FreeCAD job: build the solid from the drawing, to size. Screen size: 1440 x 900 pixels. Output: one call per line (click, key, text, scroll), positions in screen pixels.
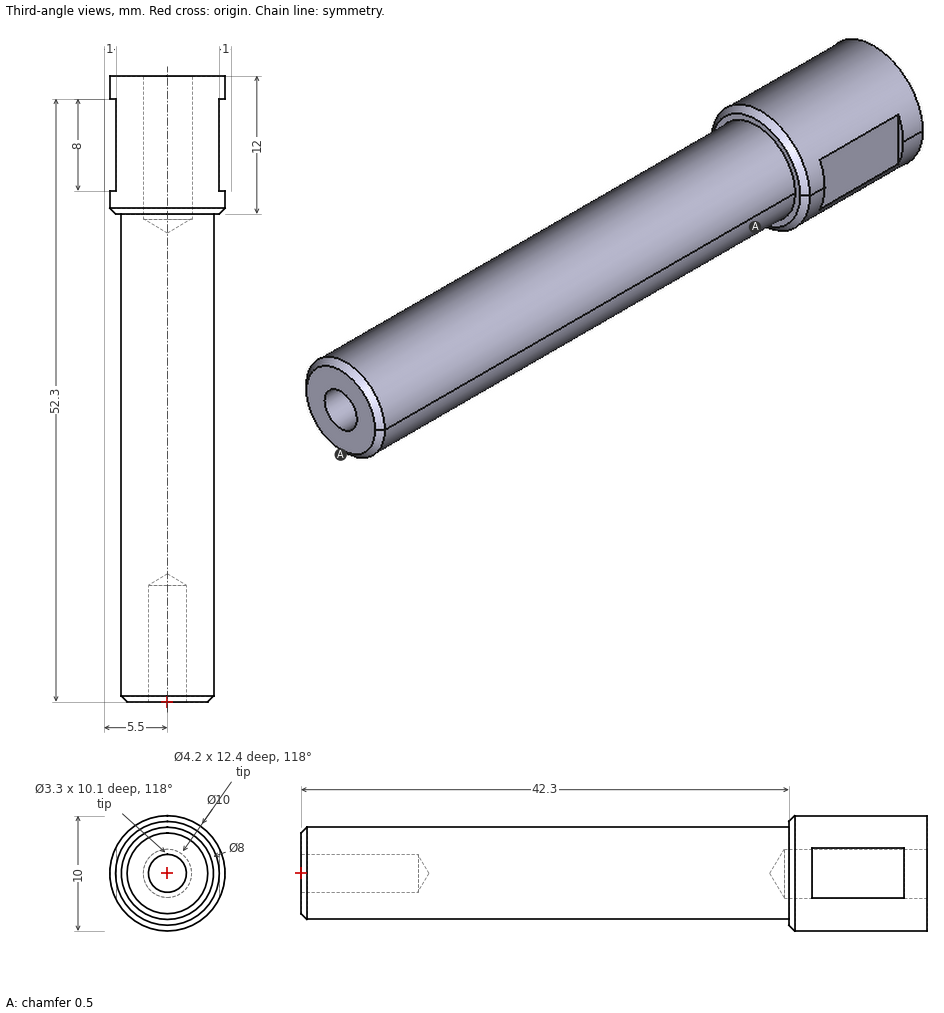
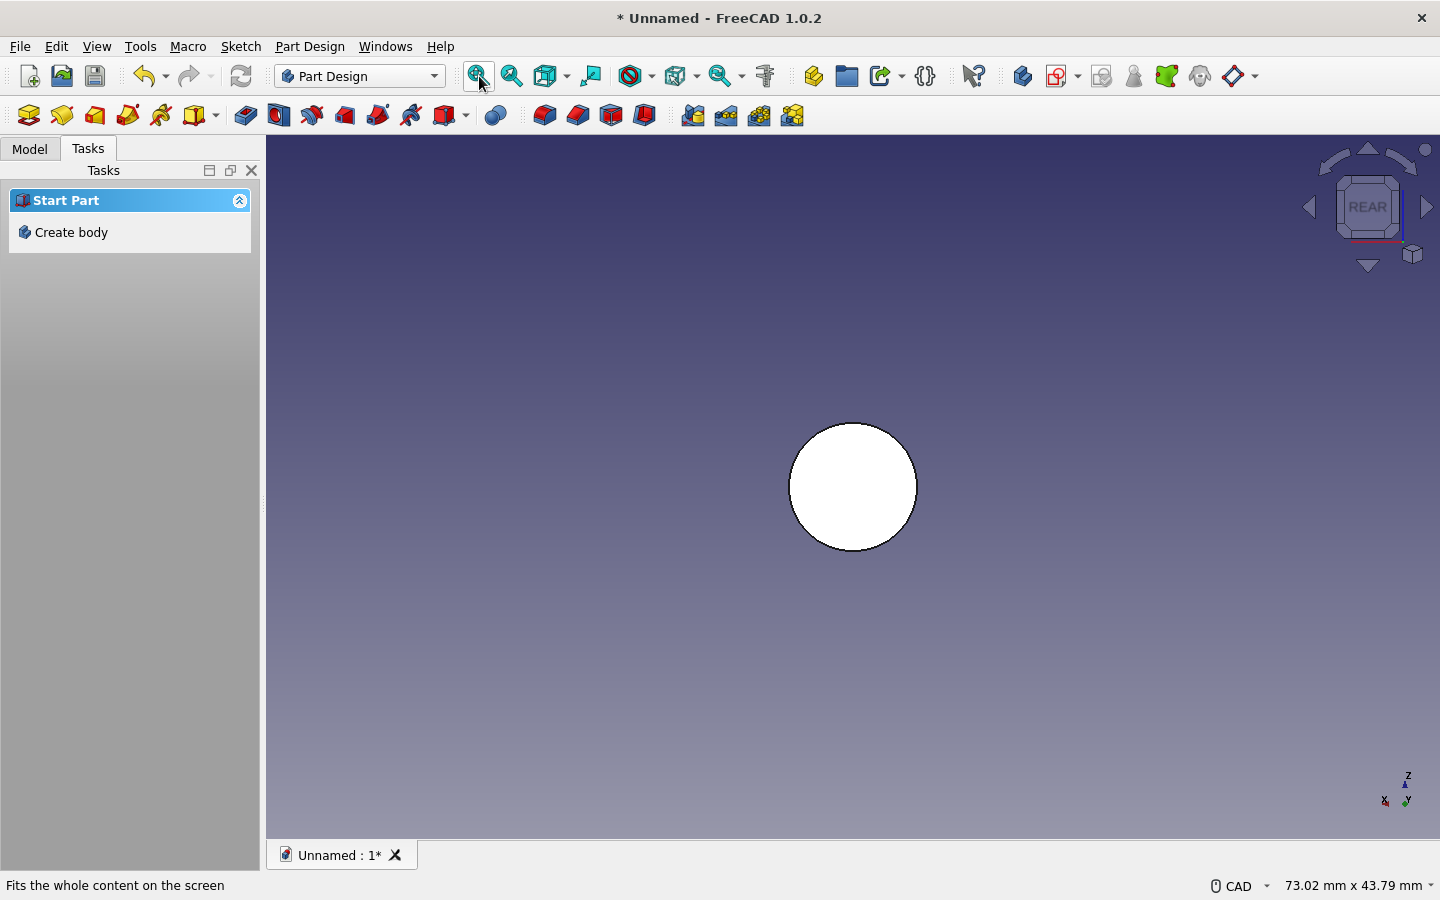
click(853, 486)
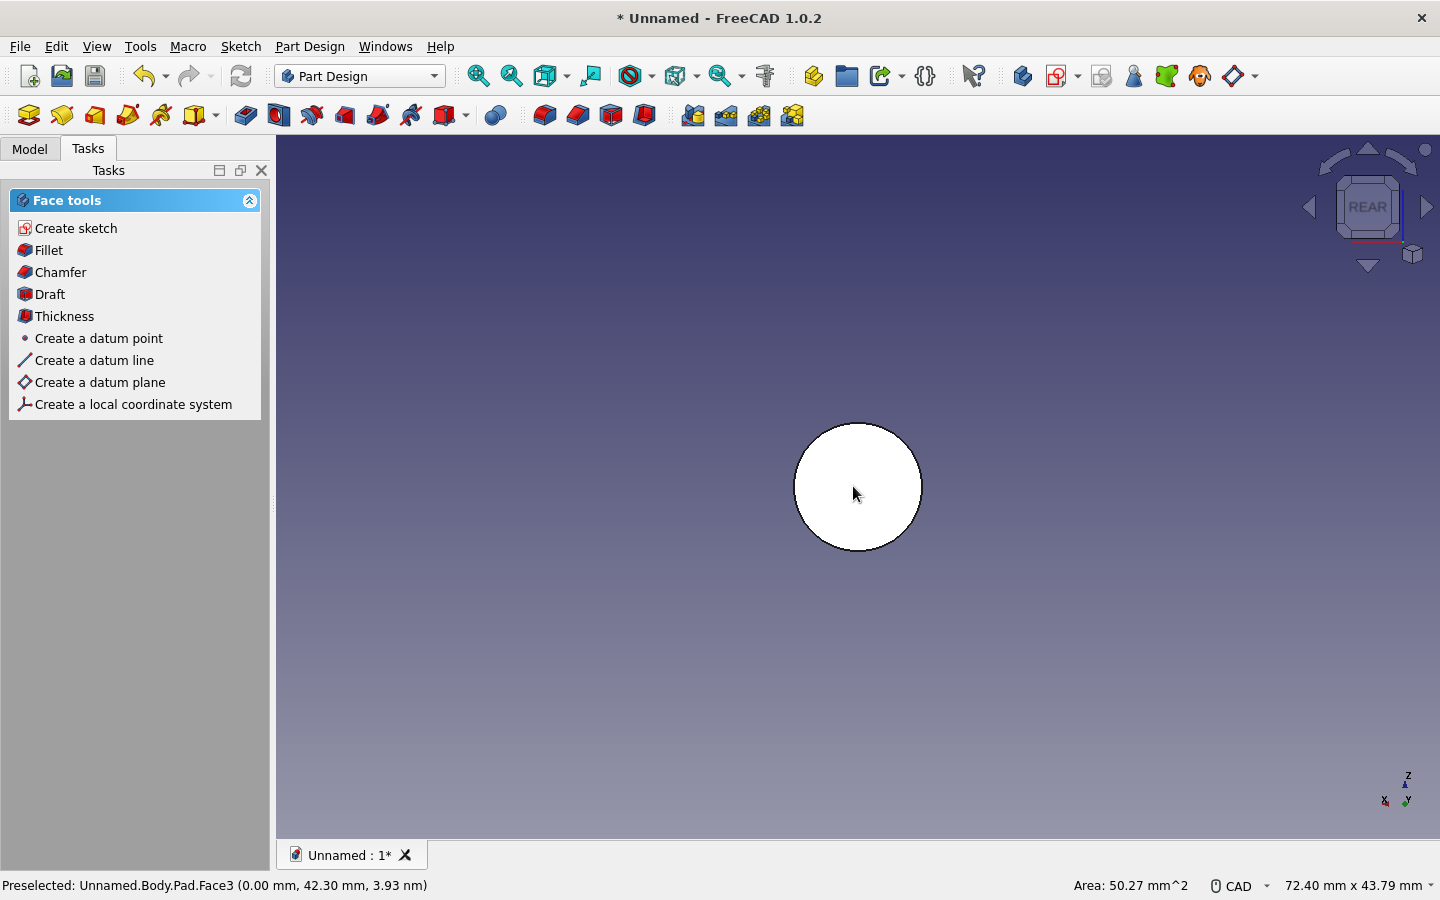
click(1056, 76)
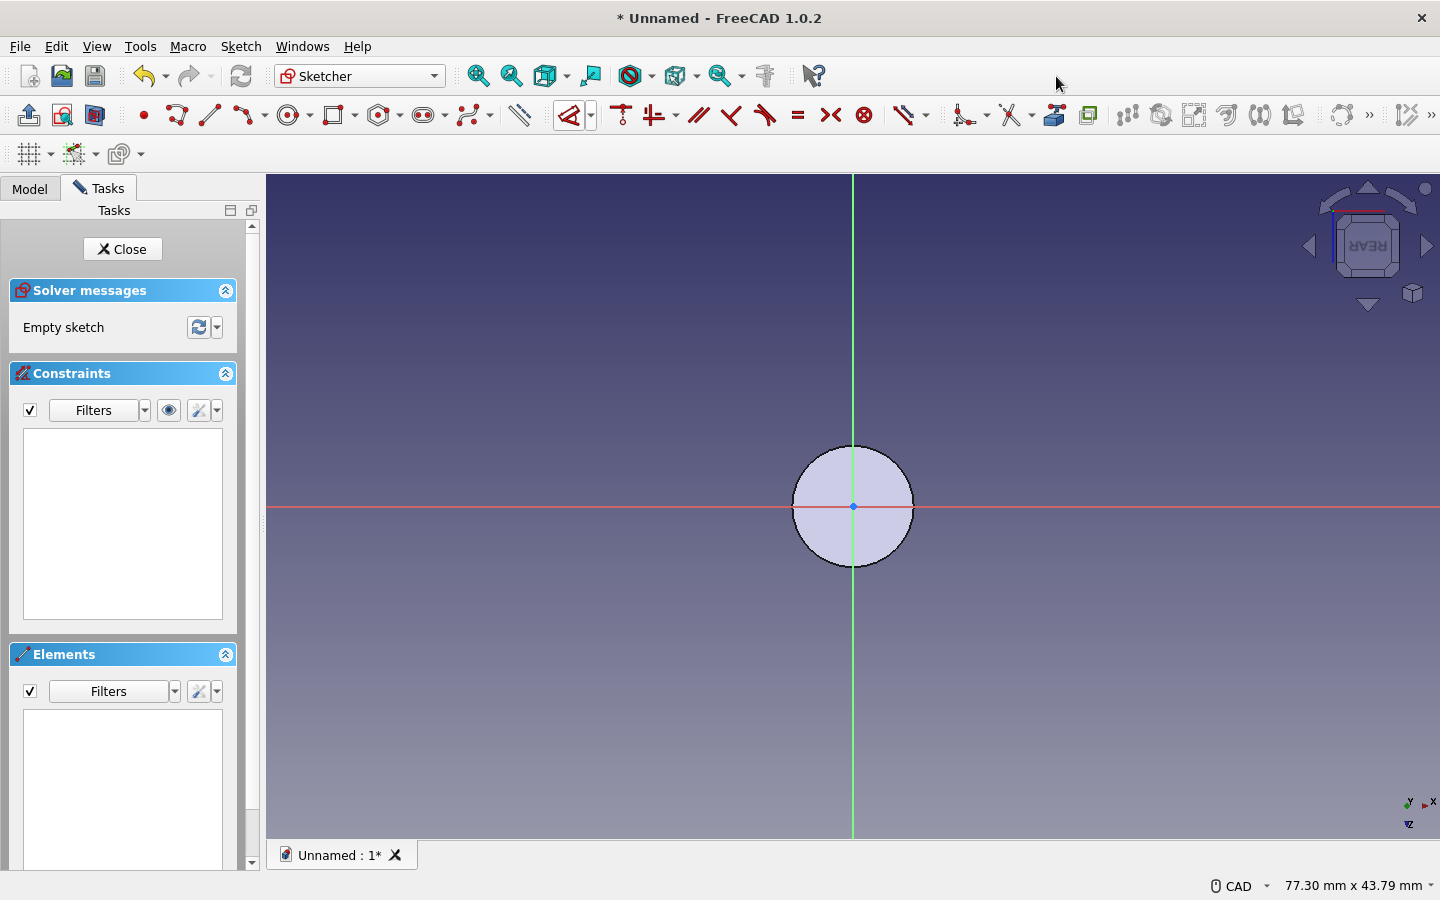
scroll(893, 506, up, 5)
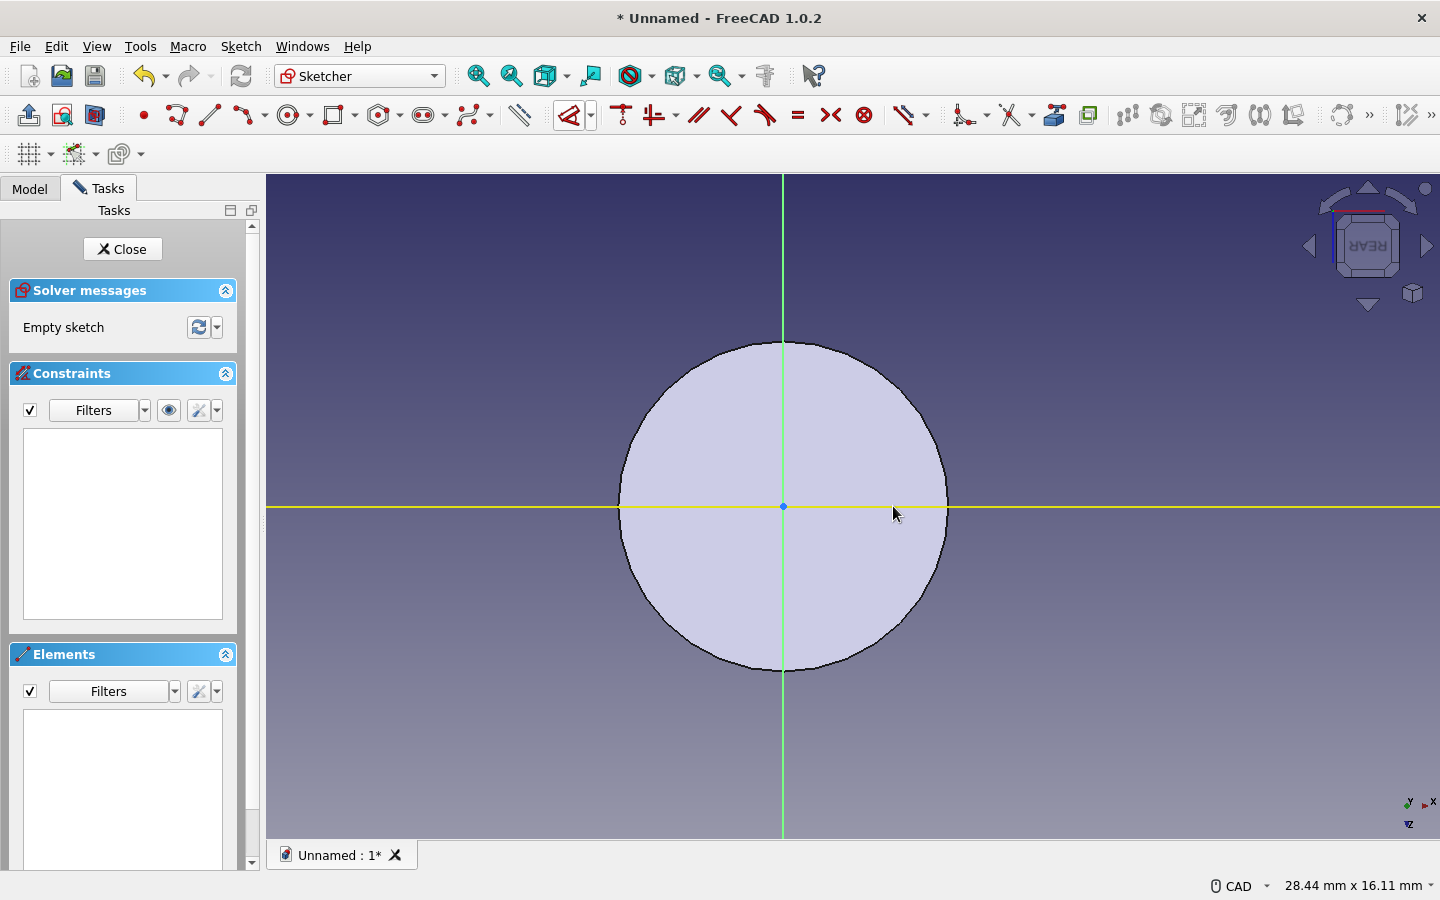
key(g)
key(c)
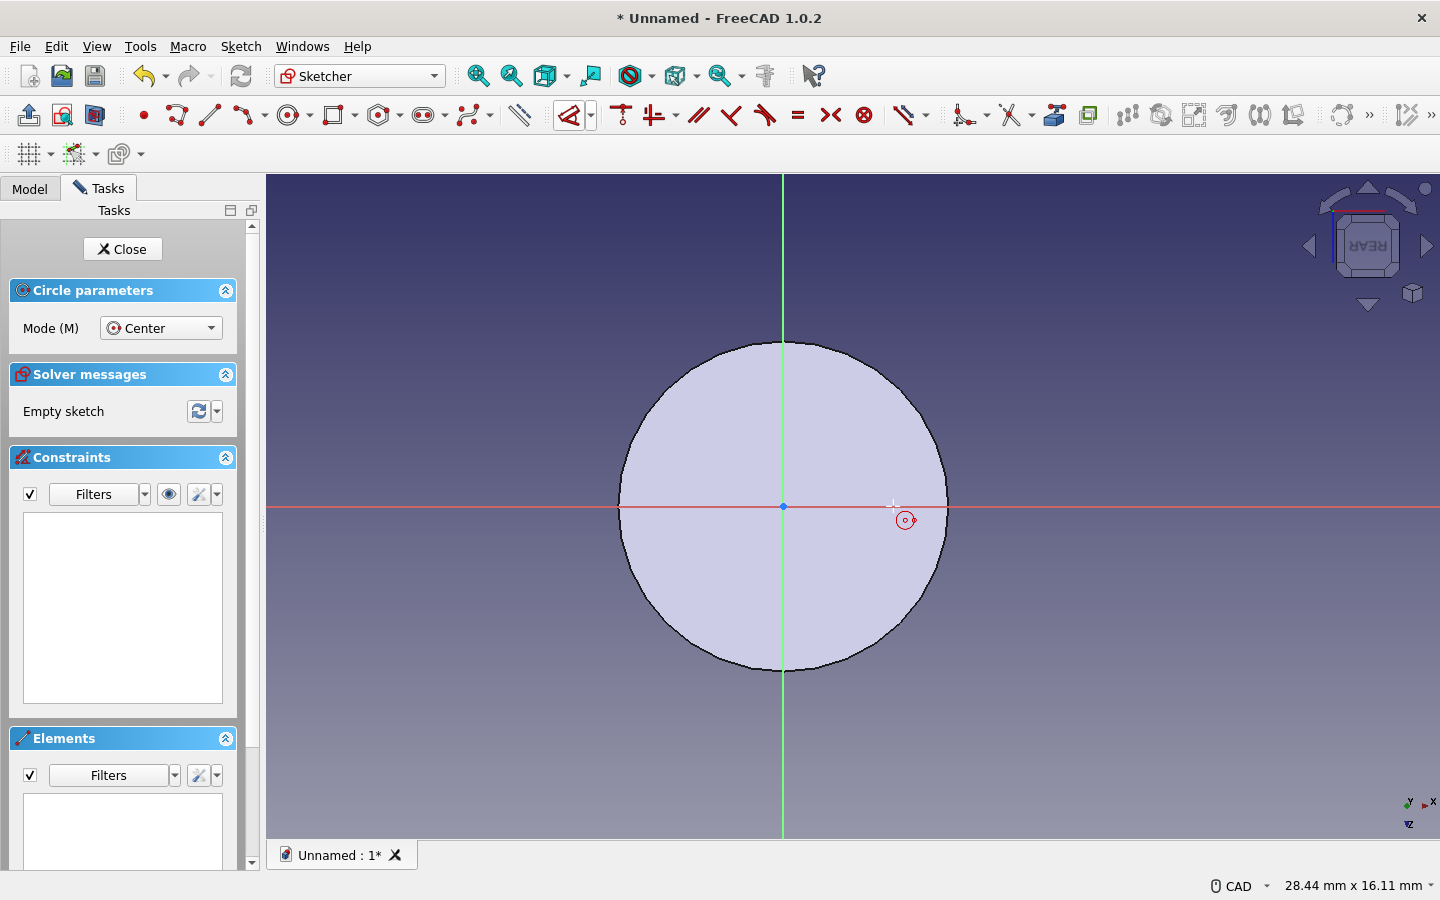
click(783, 506)
move(929, 361)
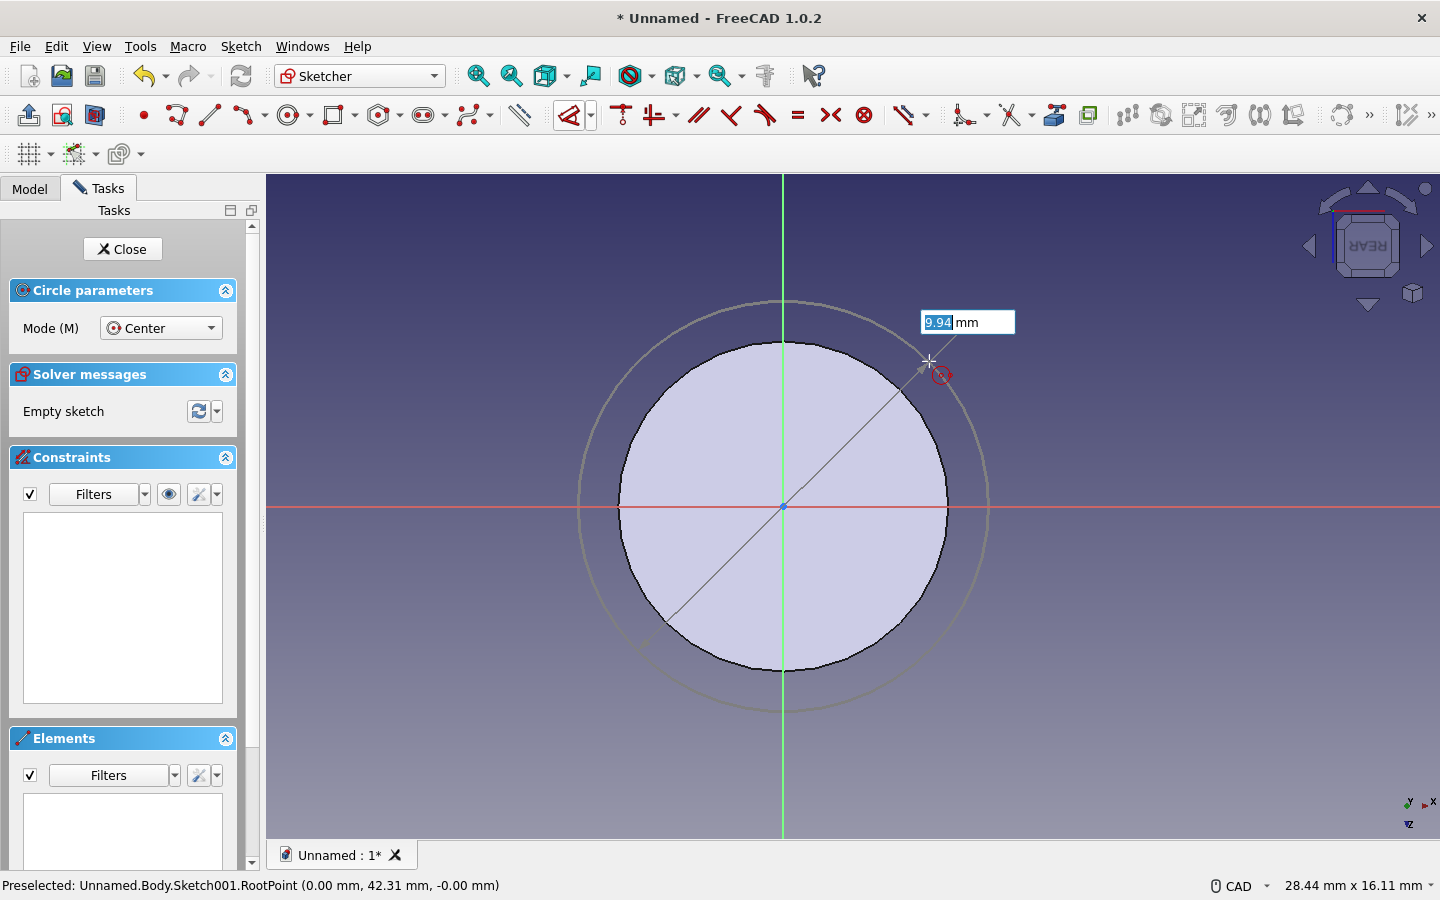
text(10)
key(Return)
key(Escape)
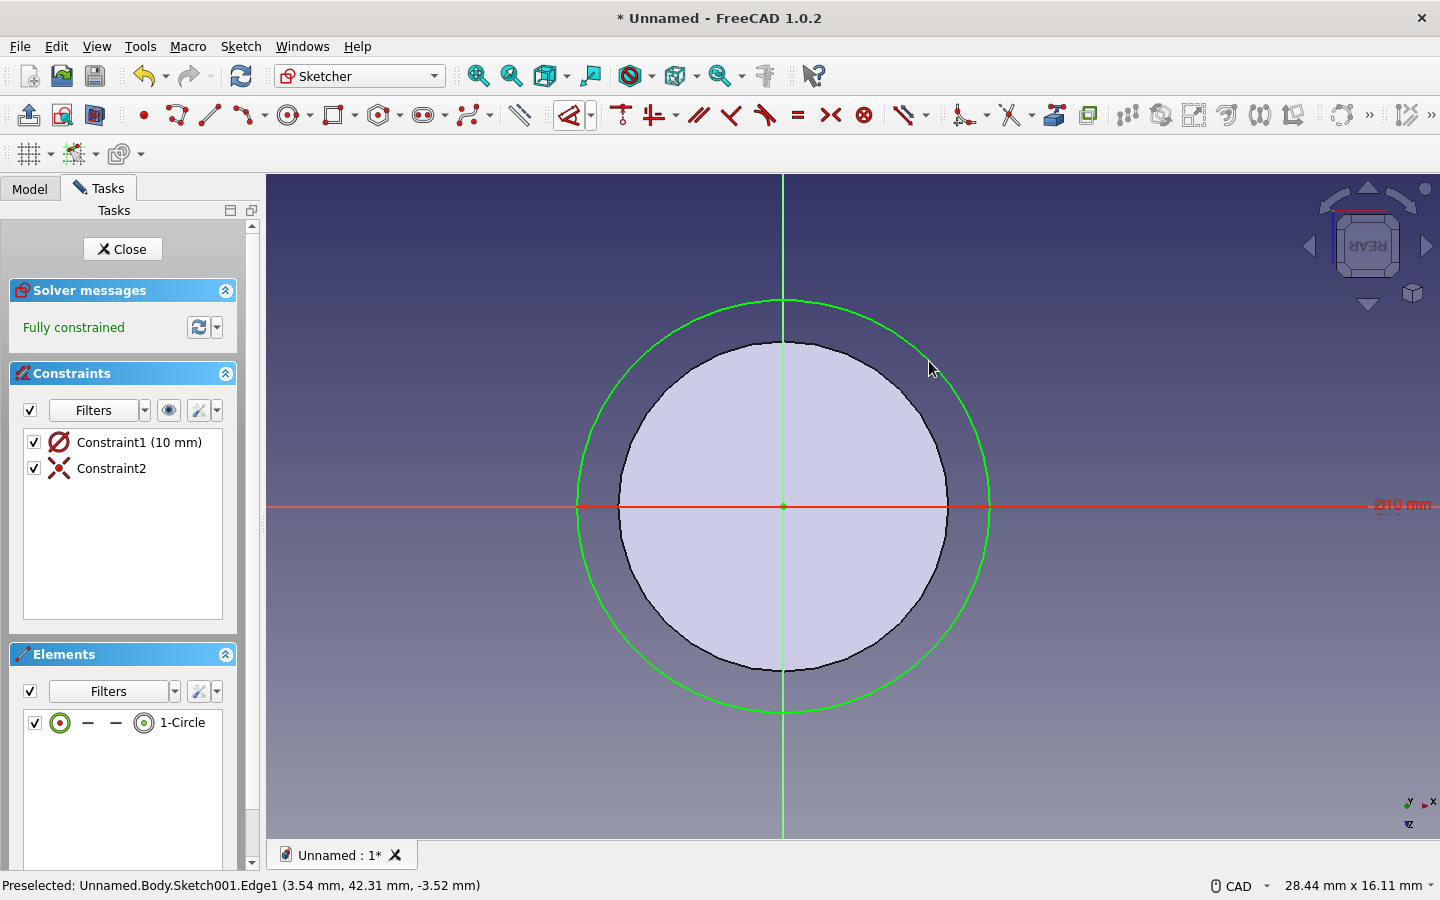
click(123, 249)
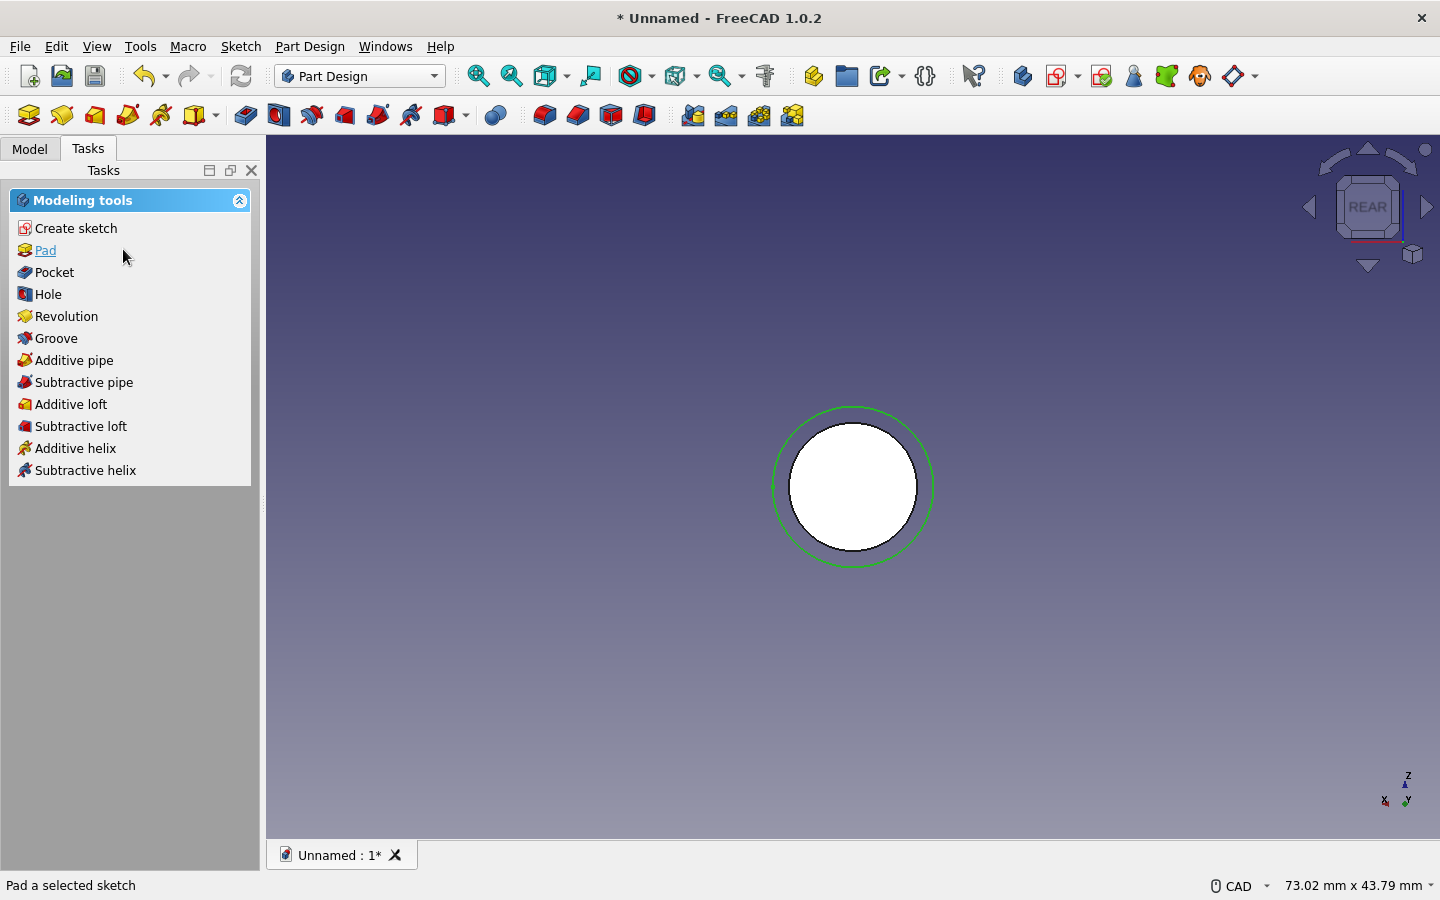
click(29, 116)